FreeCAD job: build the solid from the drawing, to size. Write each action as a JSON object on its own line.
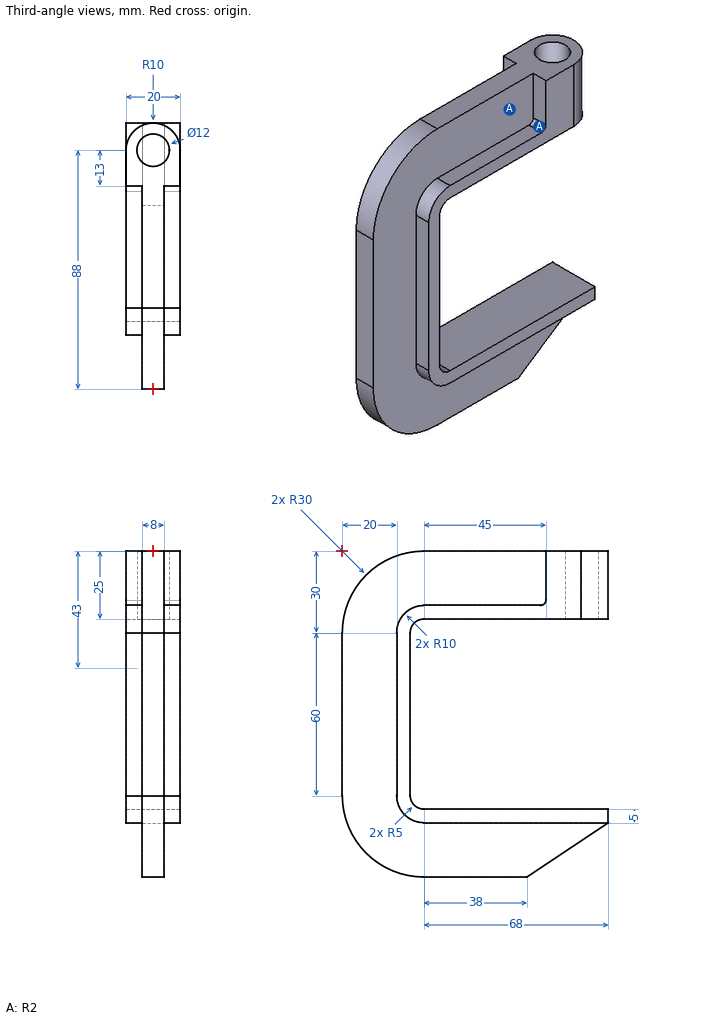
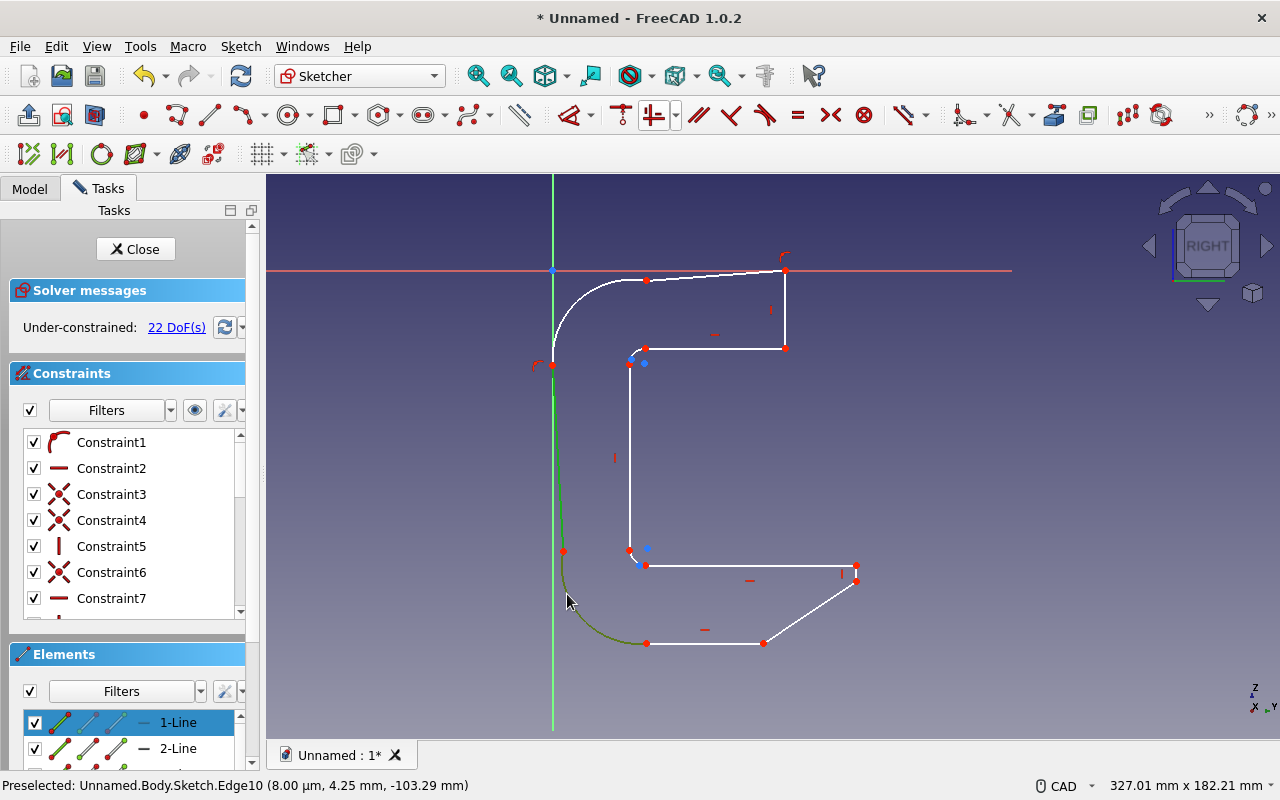
{"action": "key", "text": "t"}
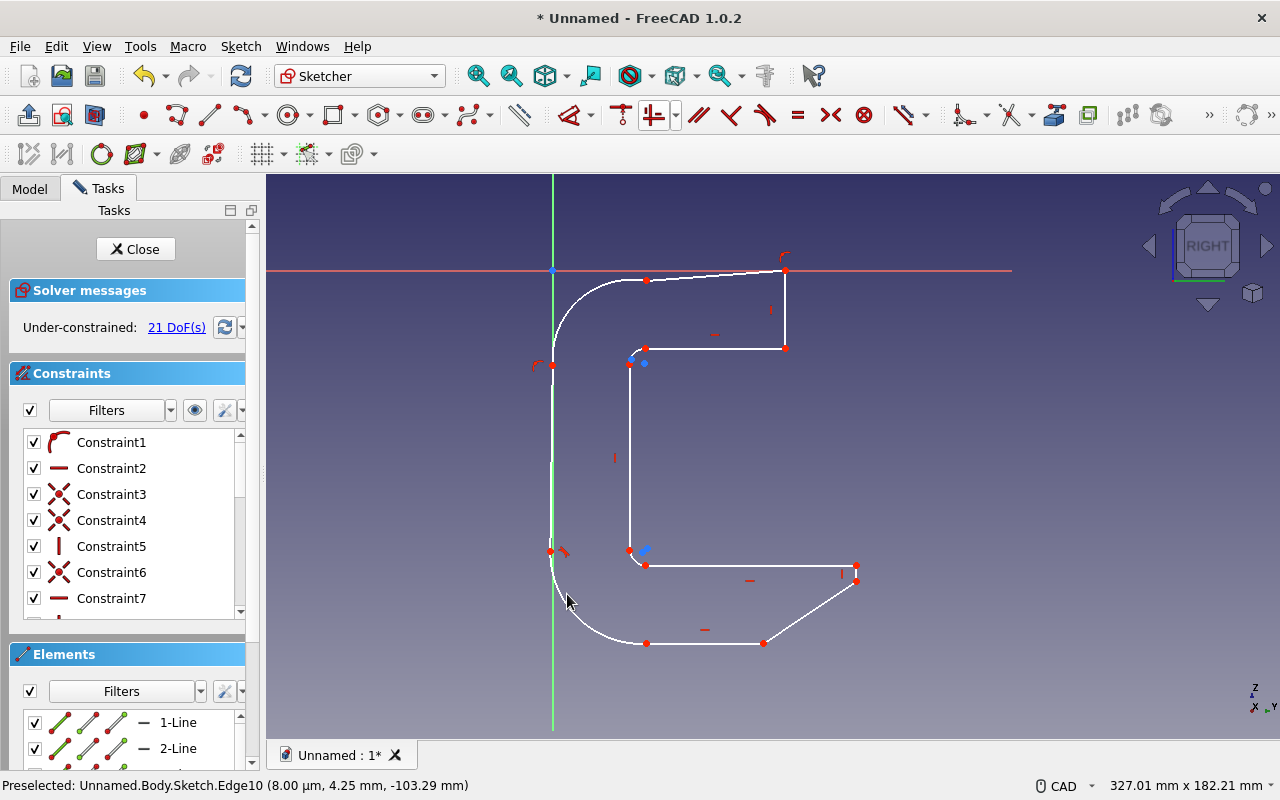
{"action": "left_click", "coordinate": [552, 421]}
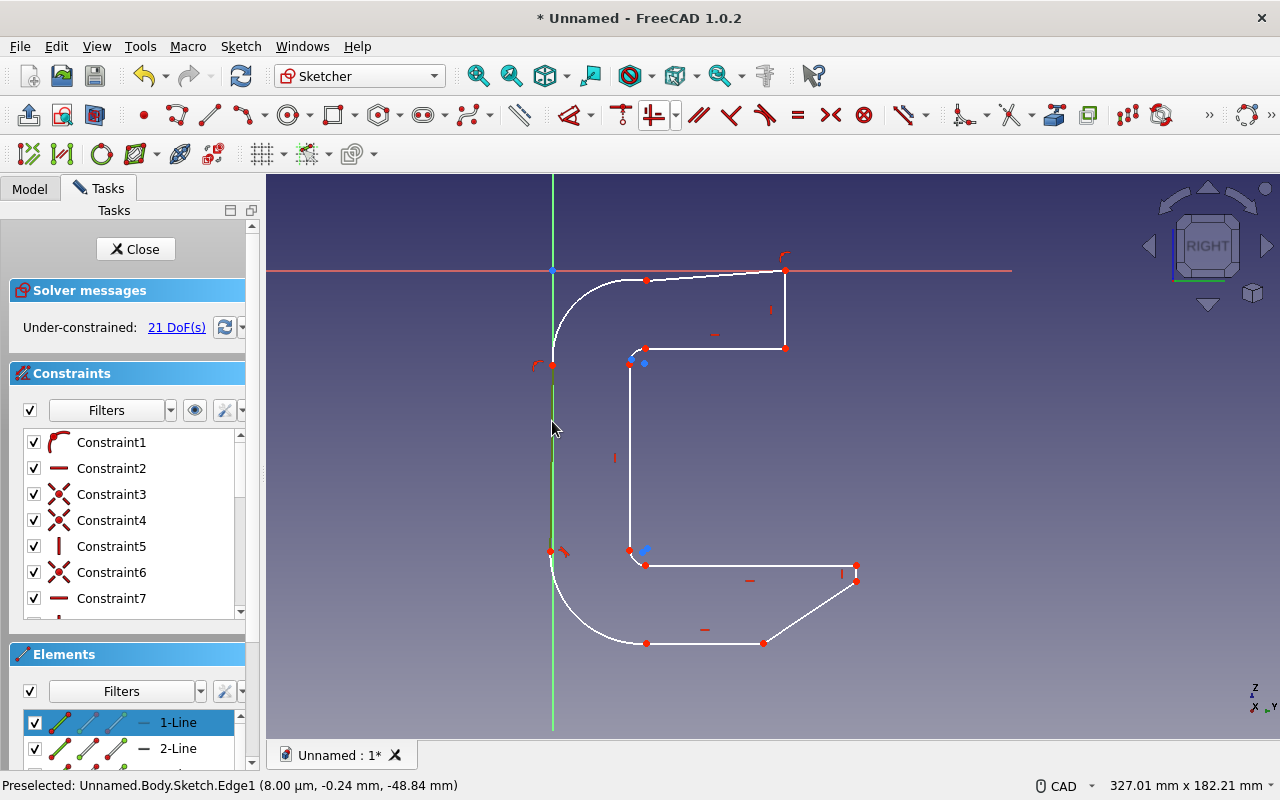
{"action": "left_click", "coordinate": [603, 285]}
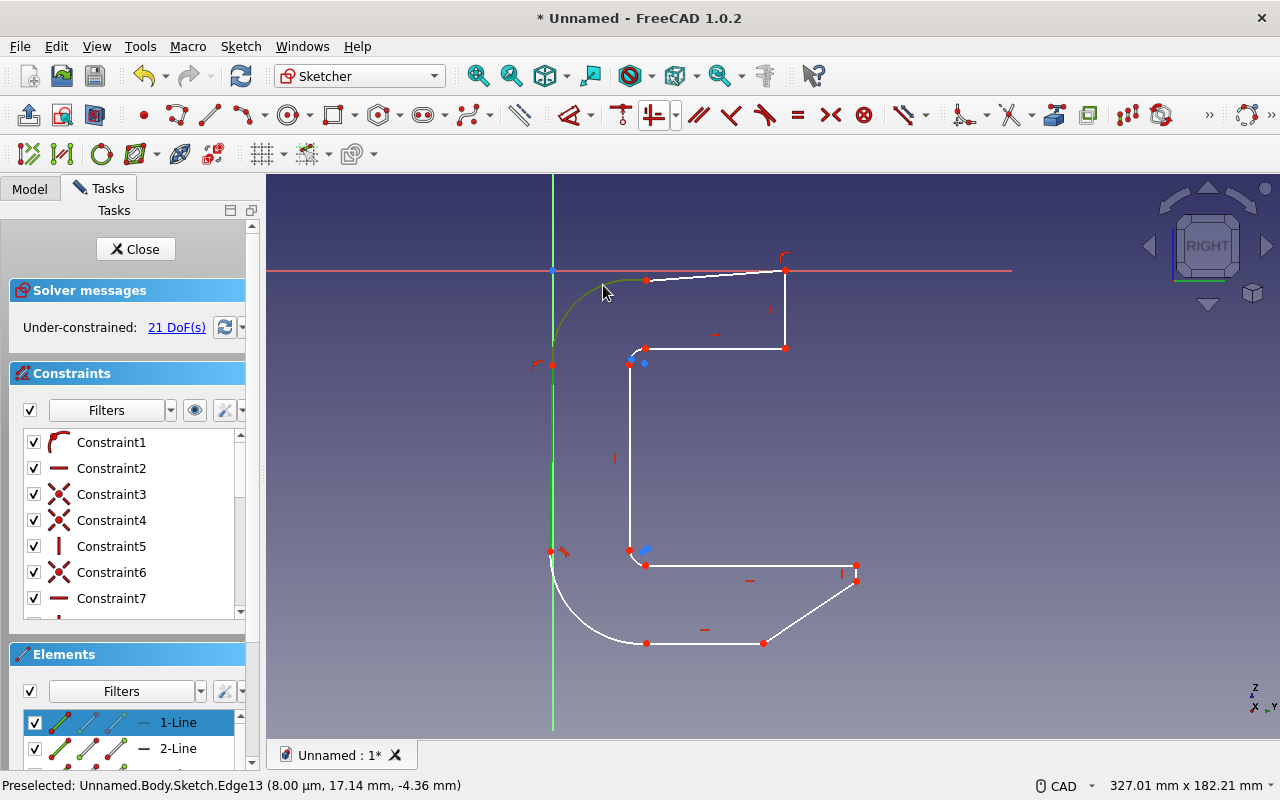
{"action": "left_click", "coordinate": [765, 116]}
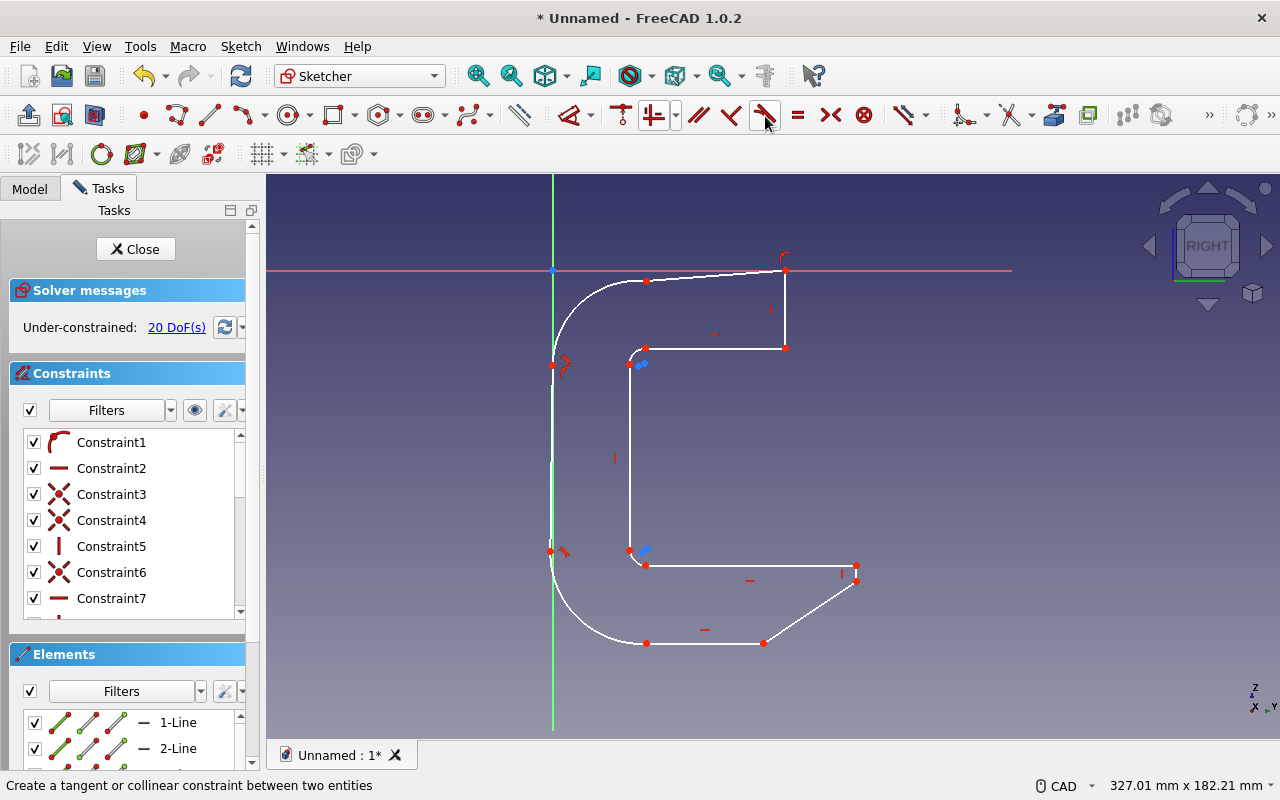
{"action": "left_click", "coordinate": [682, 644]}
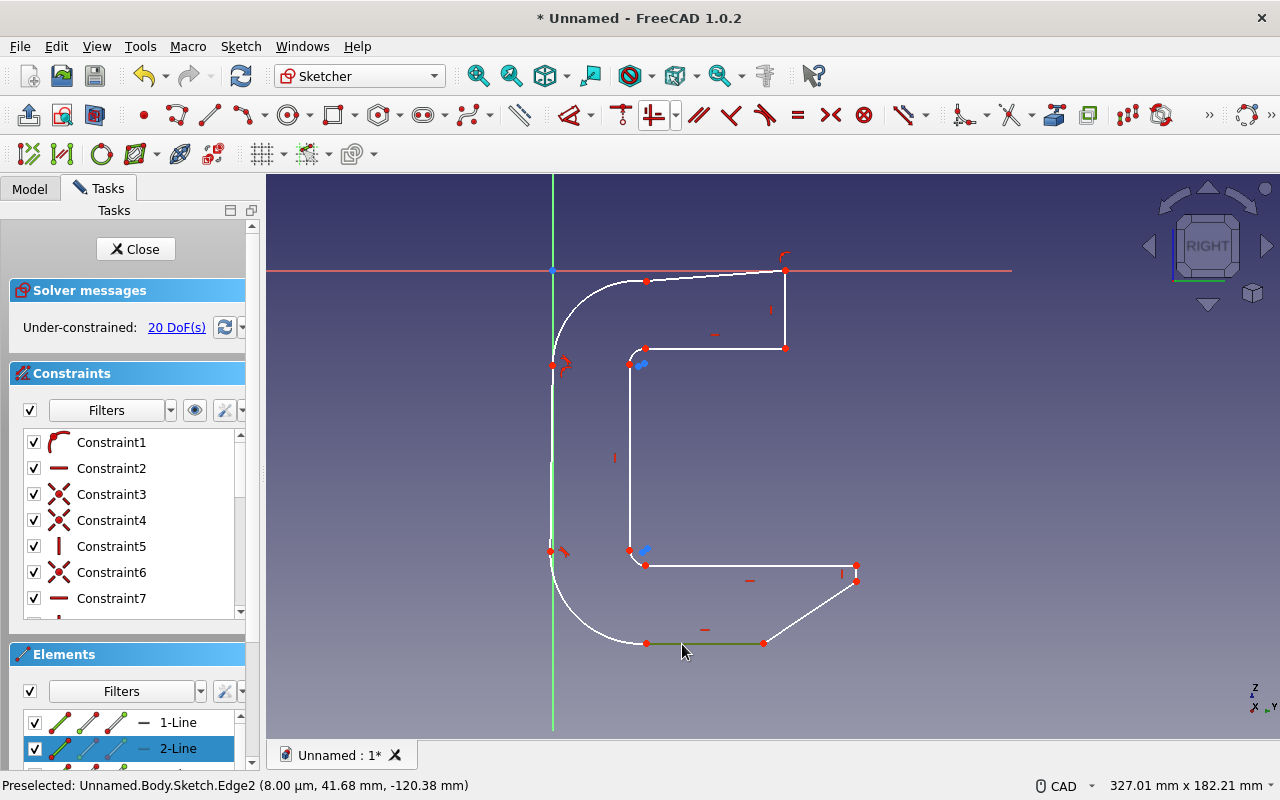
{"action": "left_click", "coordinate": [603, 635]}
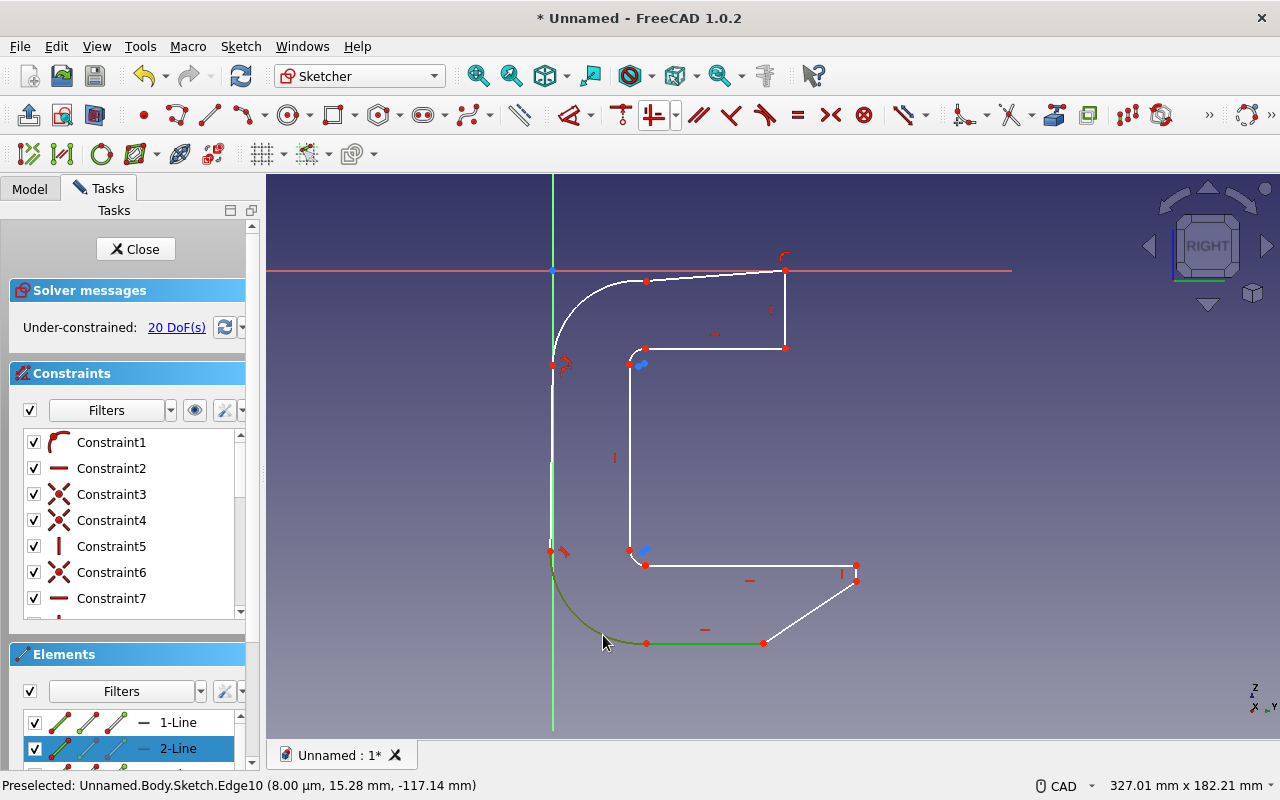
{"action": "left_click", "coordinate": [765, 116]}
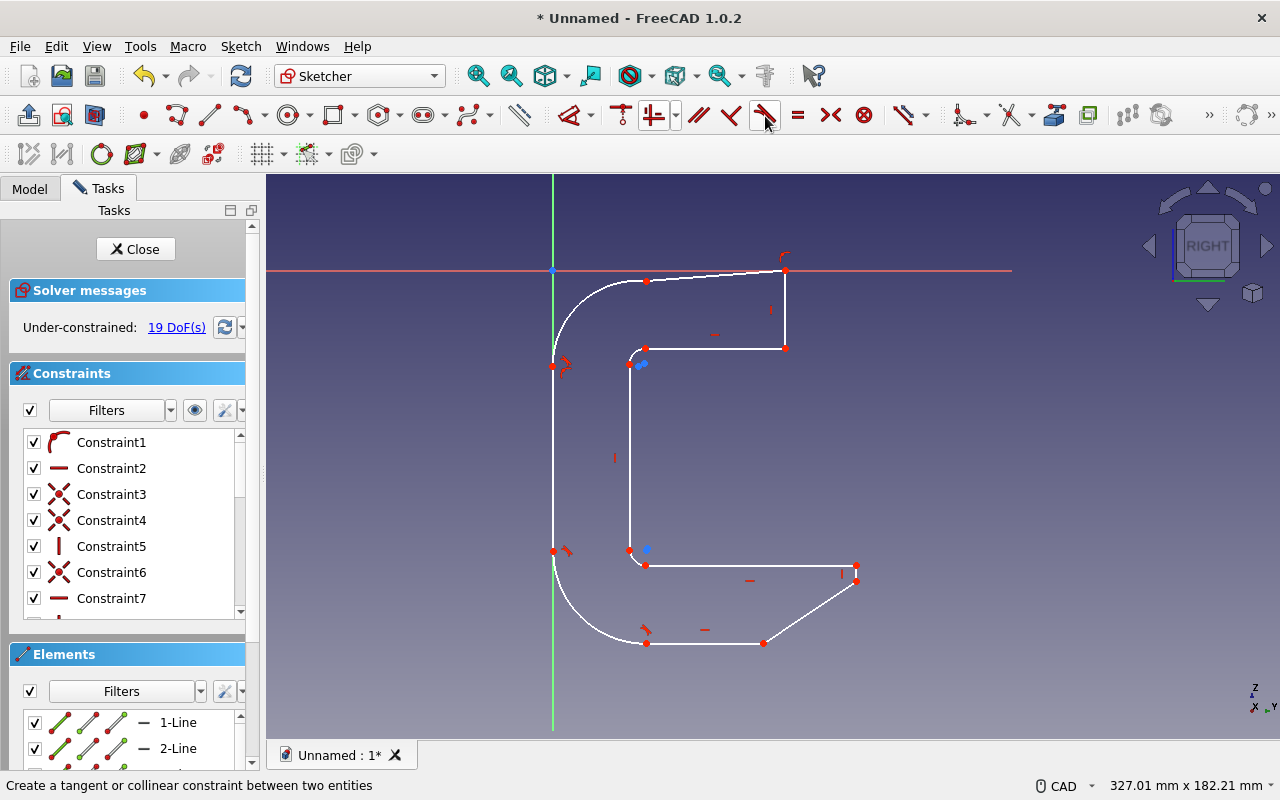
{"action": "left_click", "coordinate": [793, 566]}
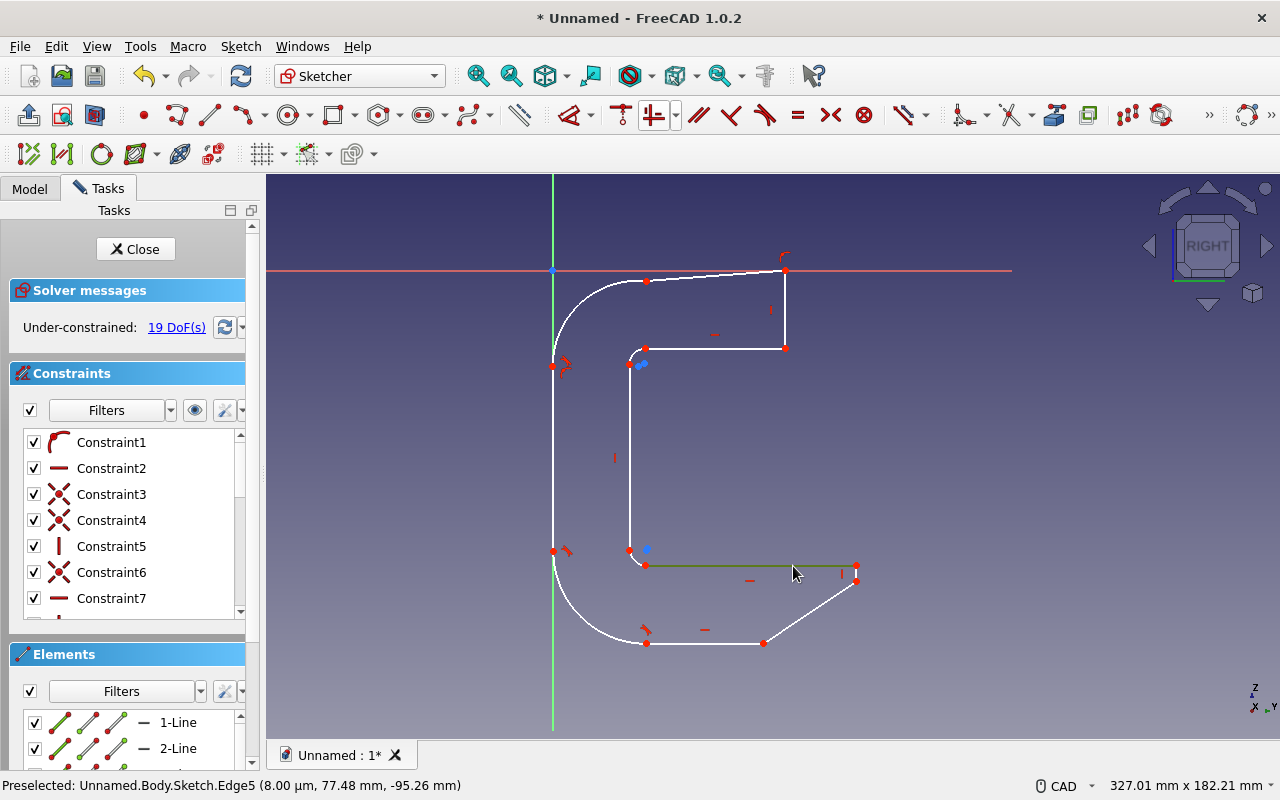
{"action": "left_click", "coordinate": [635, 561]}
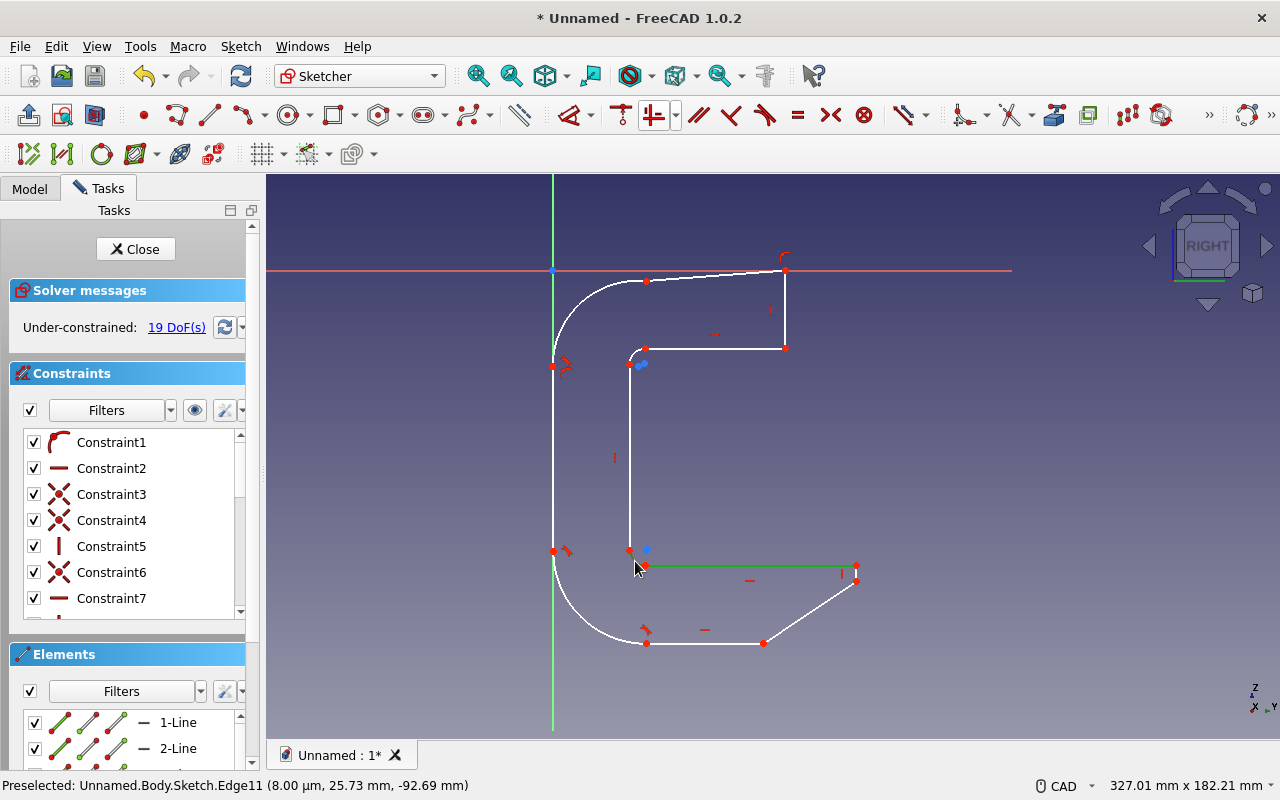
{"action": "left_click", "coordinate": [765, 116]}